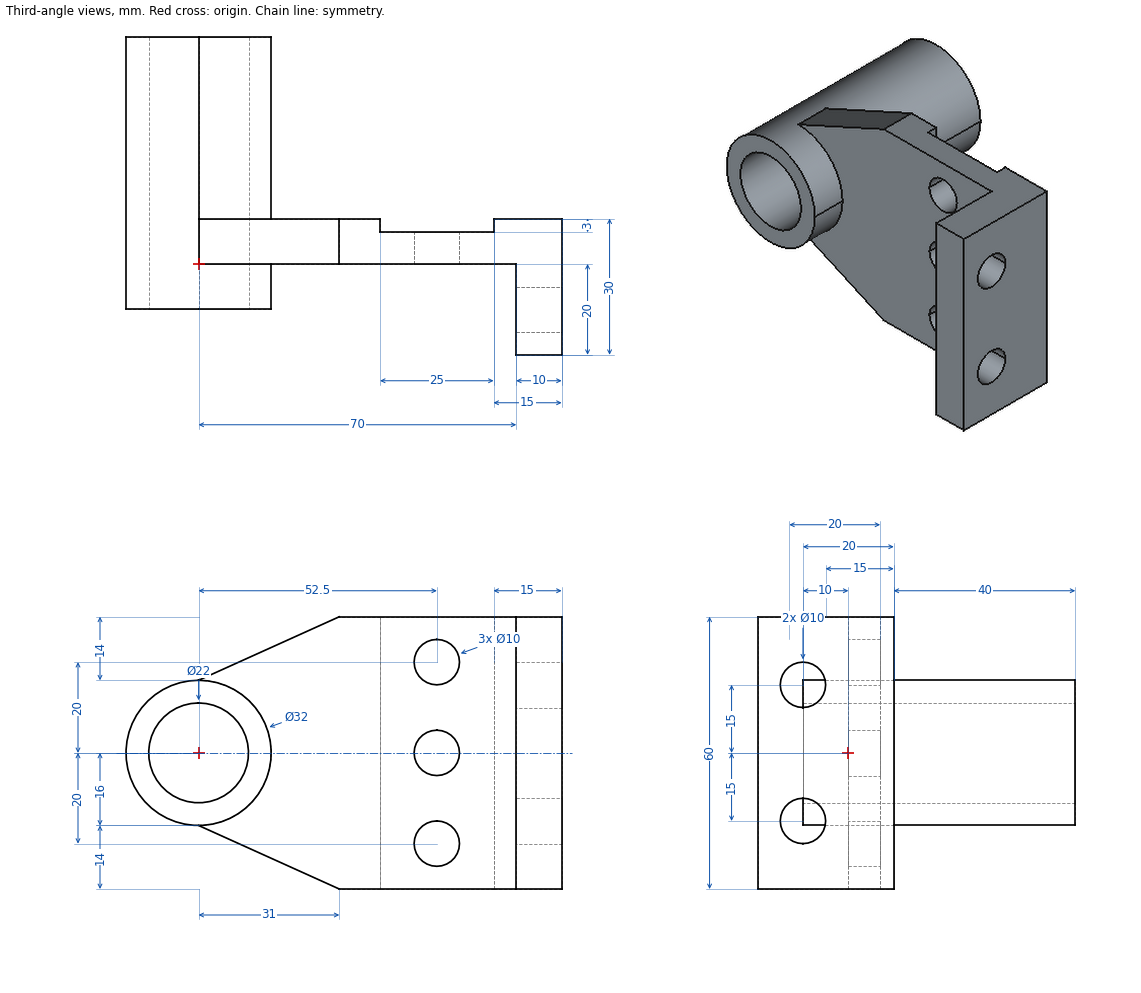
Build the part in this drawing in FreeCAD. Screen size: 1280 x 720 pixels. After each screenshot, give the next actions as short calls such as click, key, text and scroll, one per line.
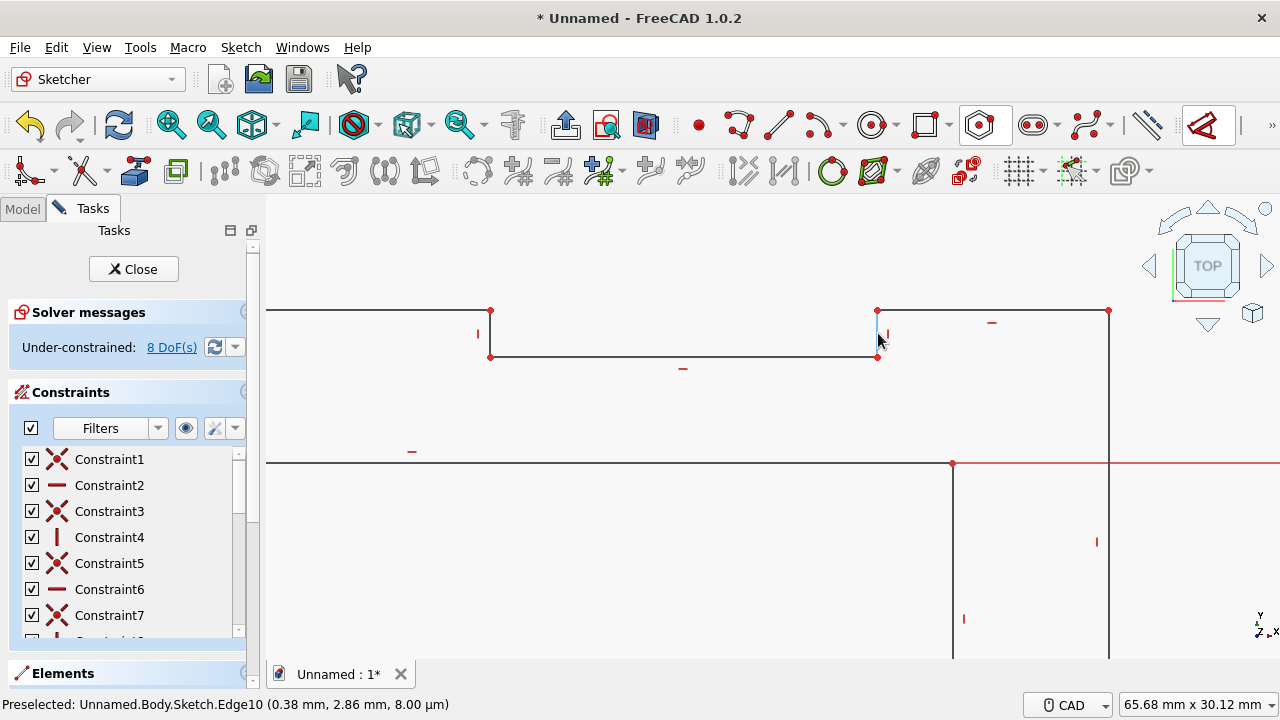
click(877, 334)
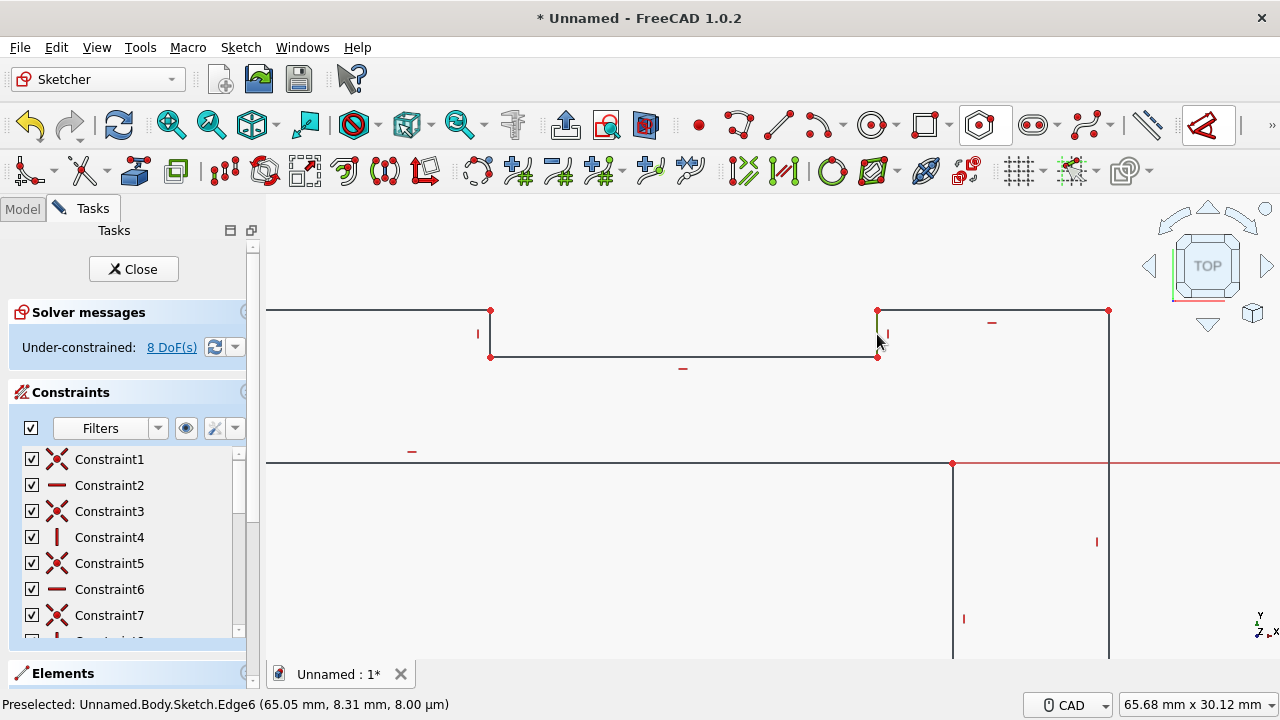
key(i)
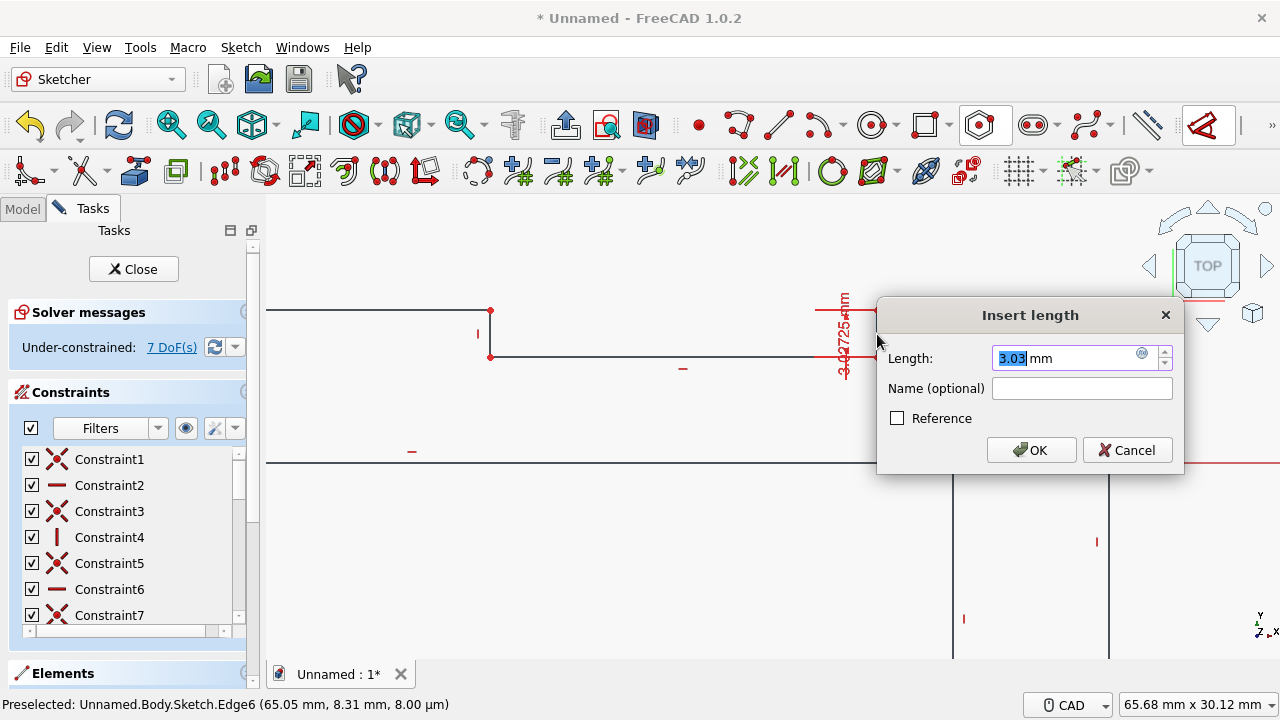
text(3)
key(Return)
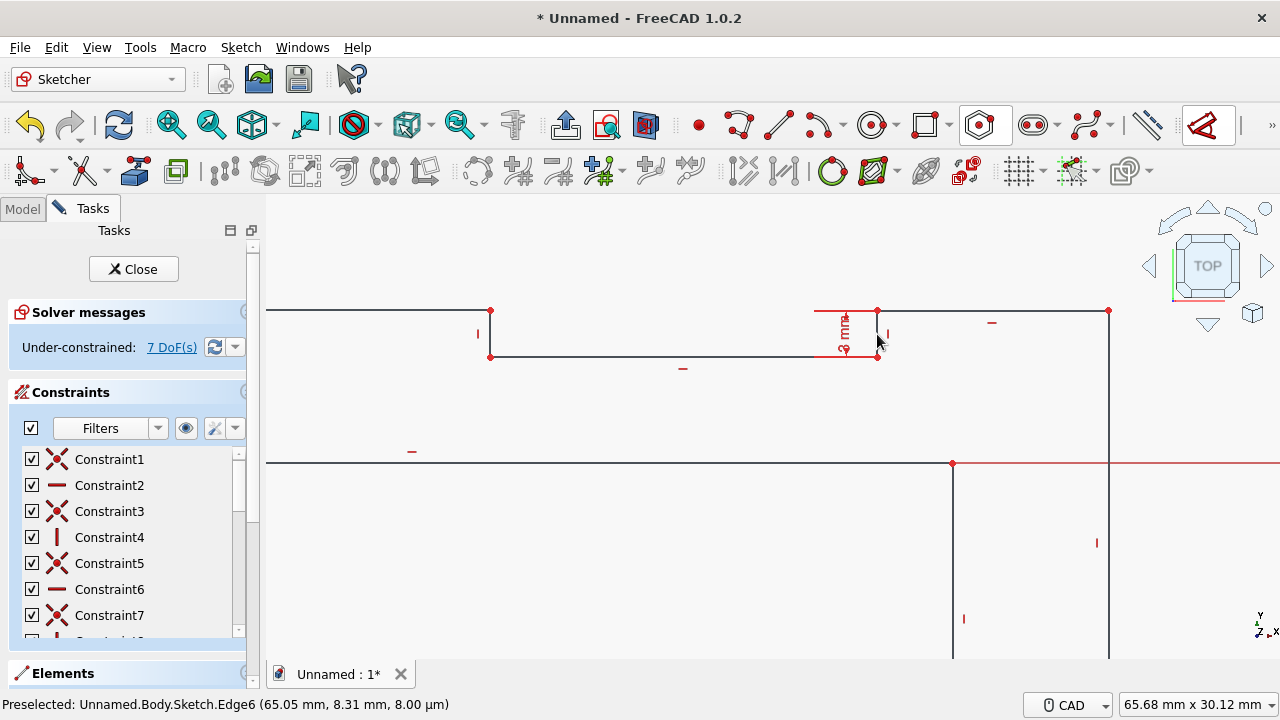
click(490, 343)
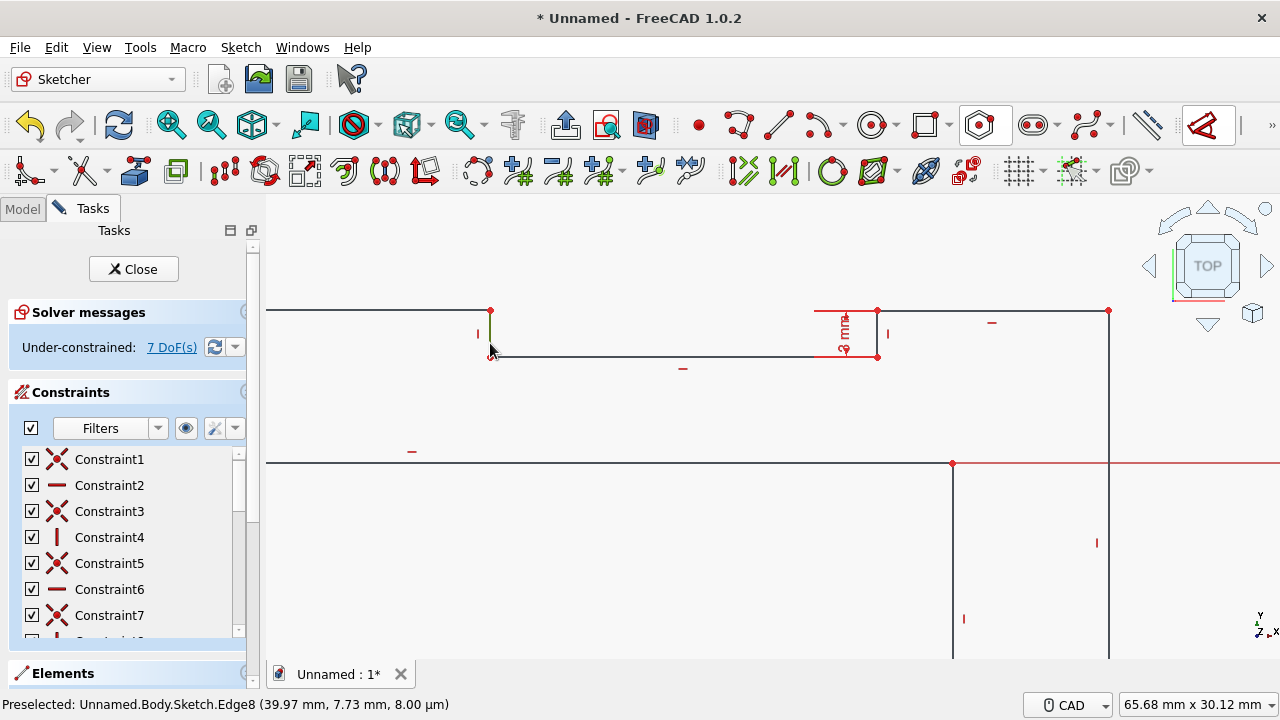
click(1230, 126)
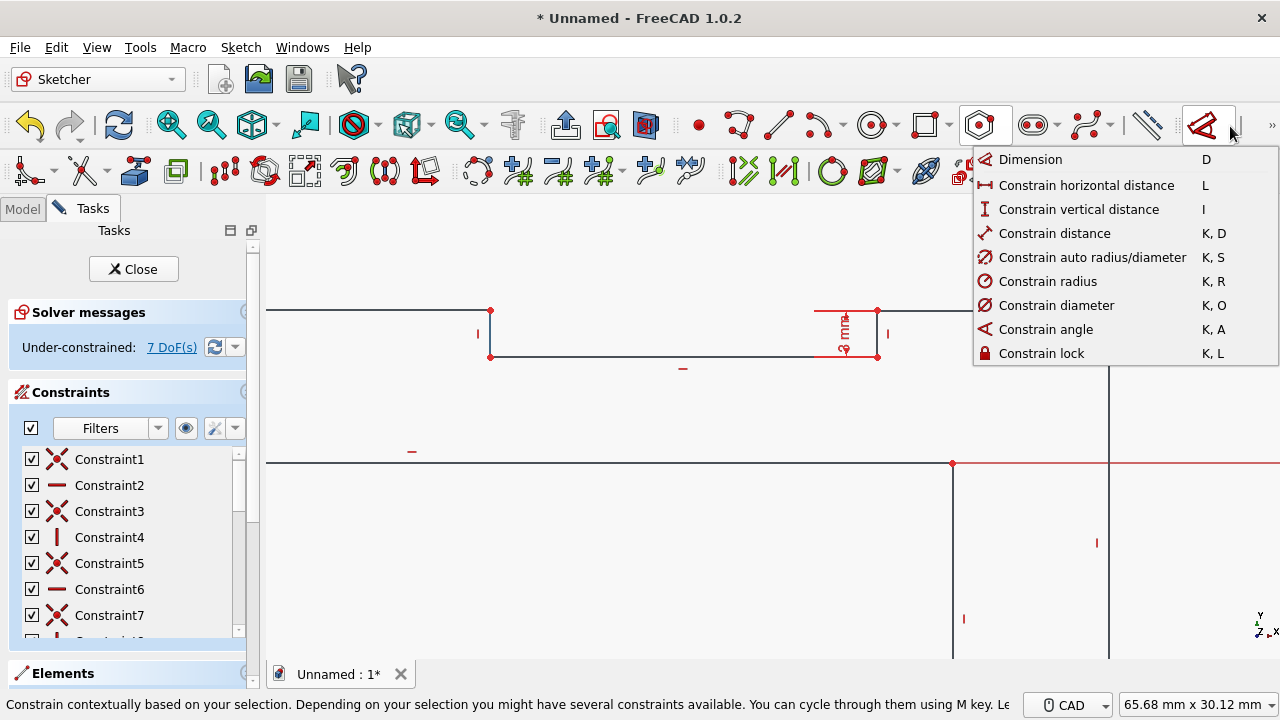
click(1126, 209)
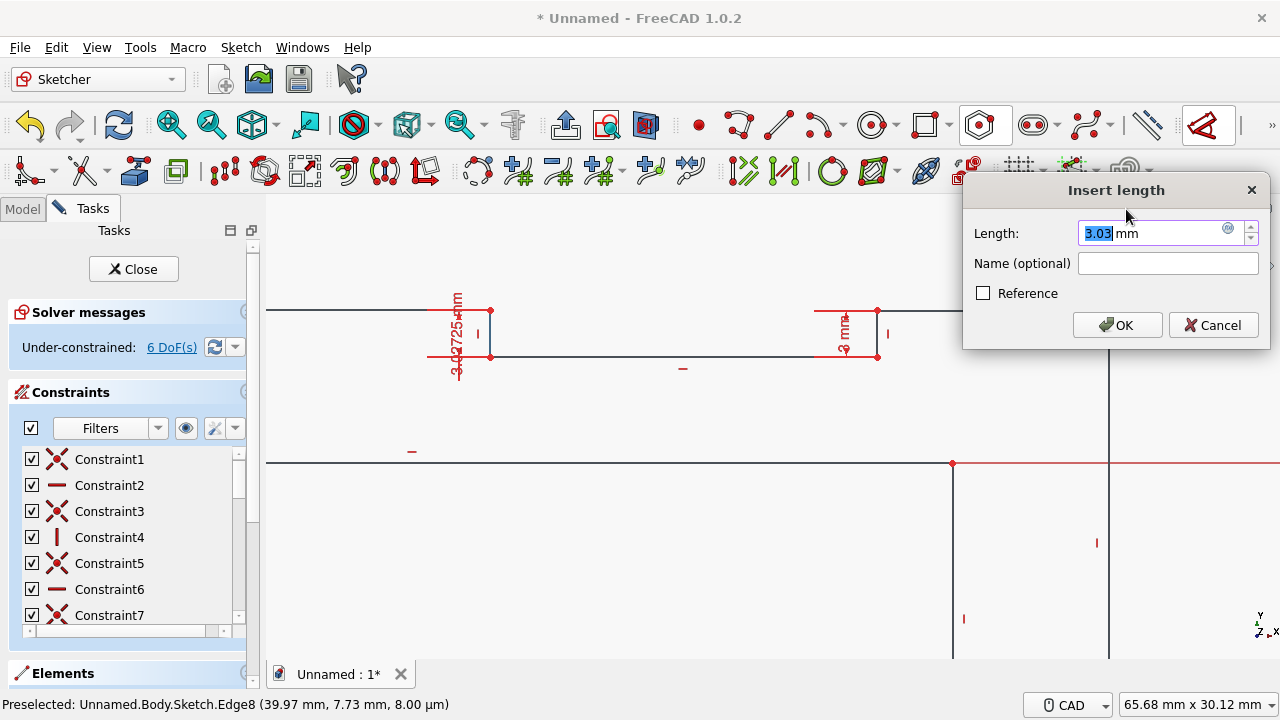
text(3)
key(Return)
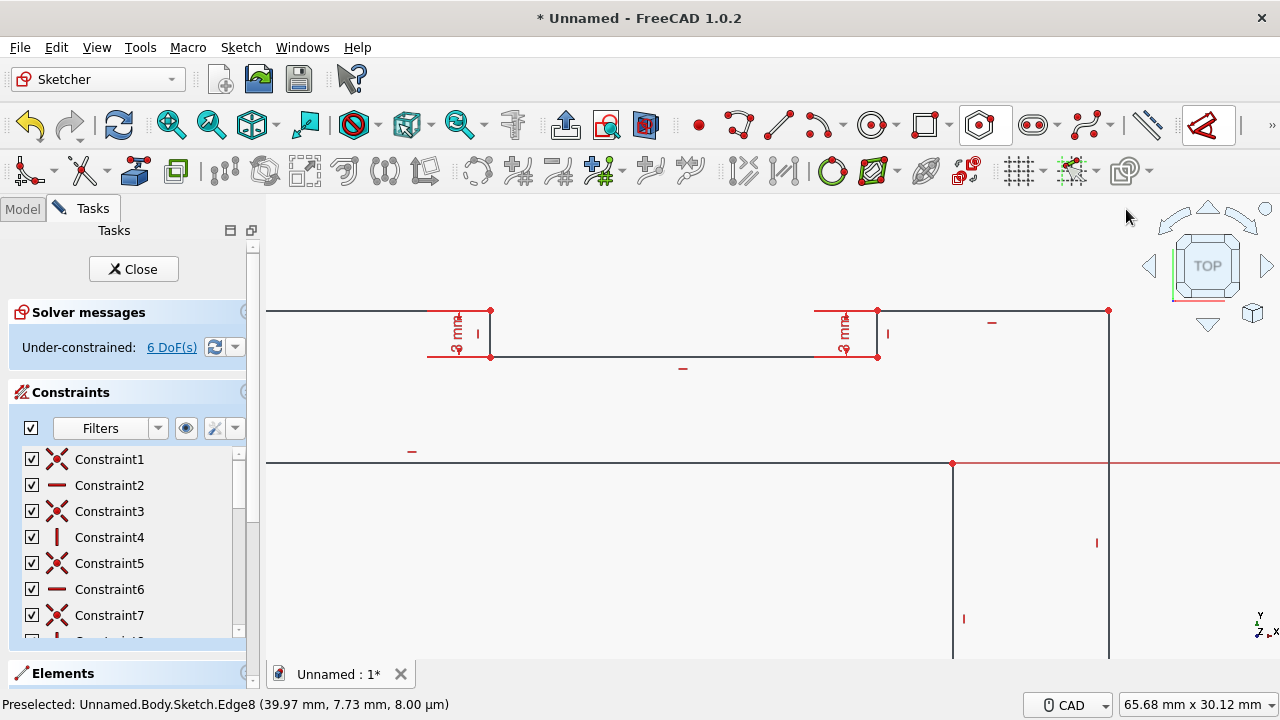
click(629, 463)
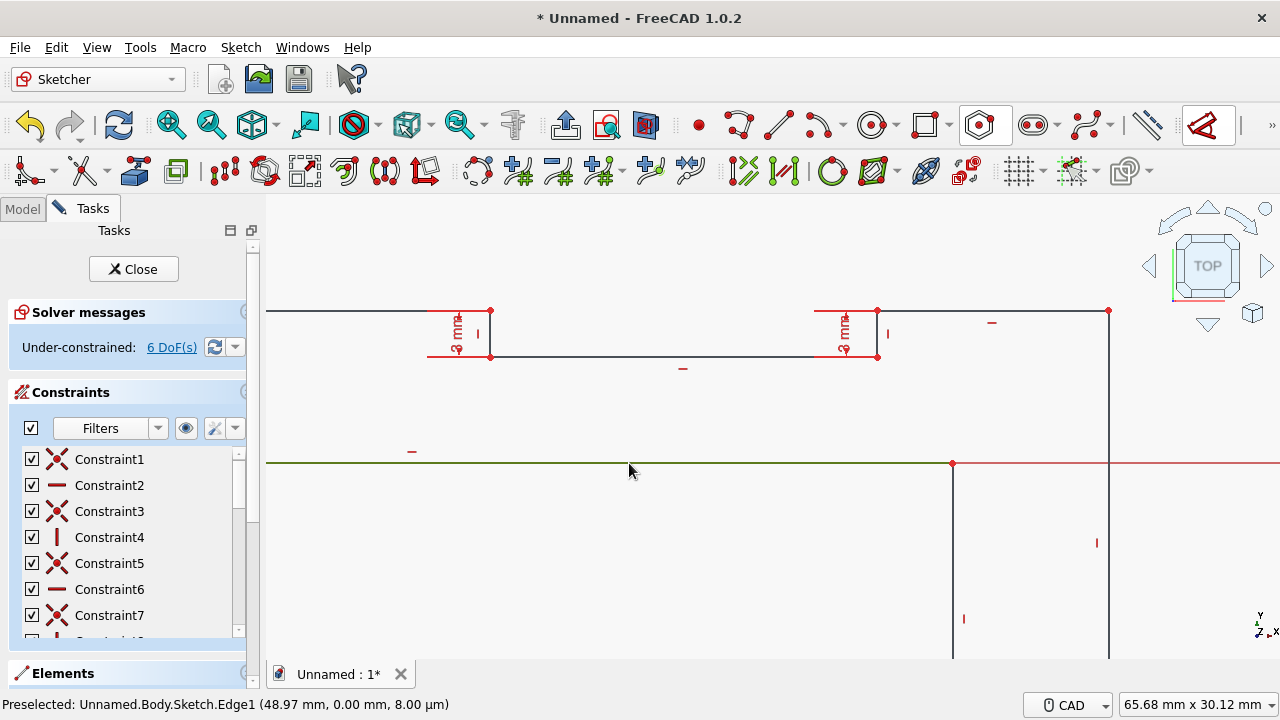
click(1230, 126)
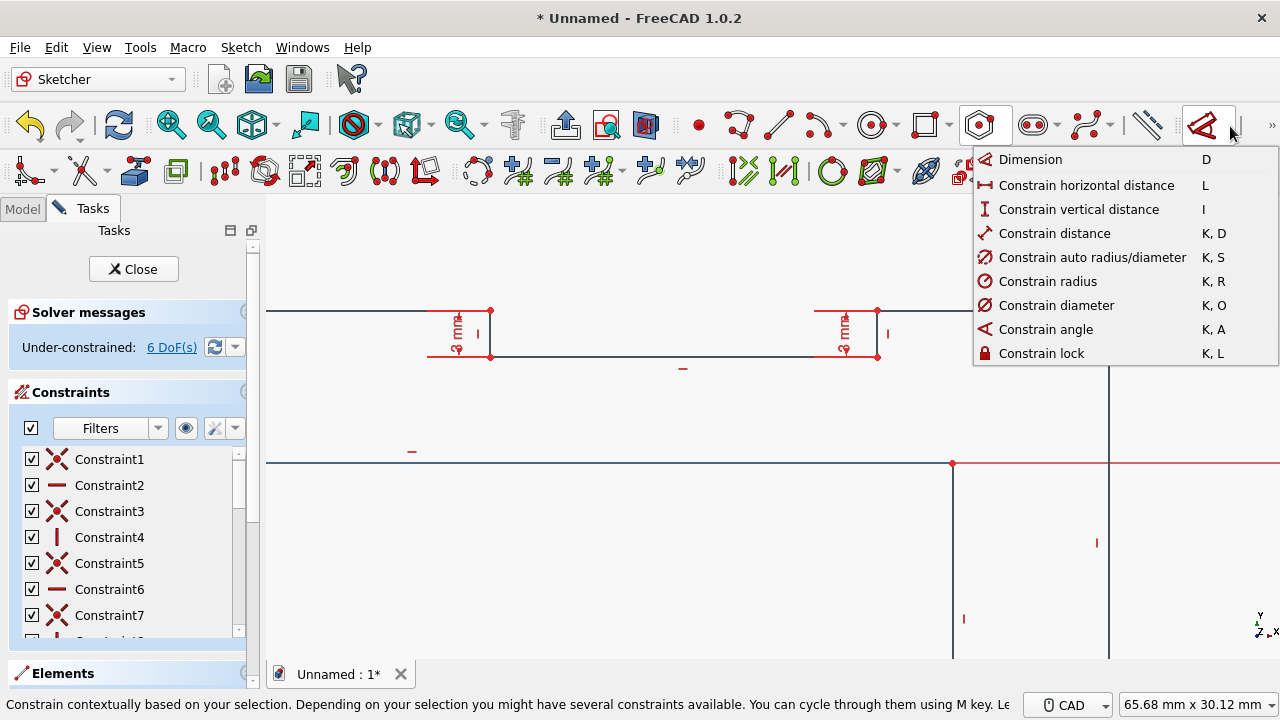
click(1126, 185)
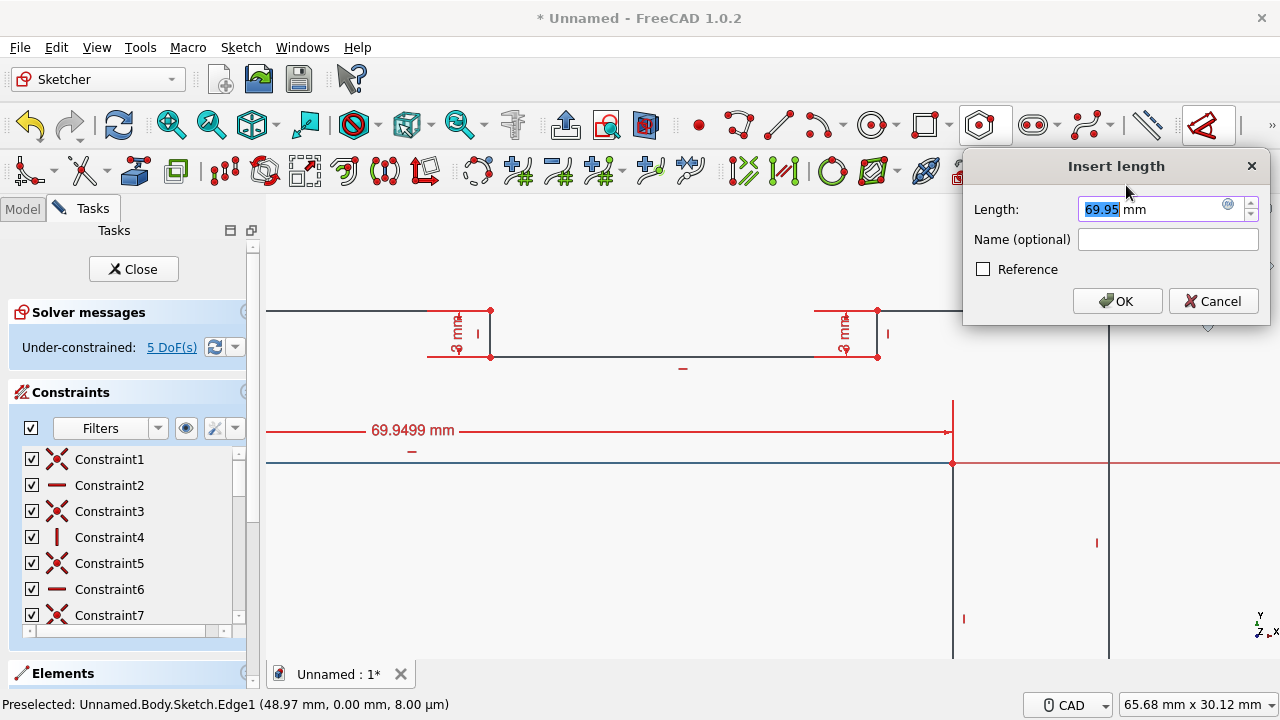
text(70)
key(Return)